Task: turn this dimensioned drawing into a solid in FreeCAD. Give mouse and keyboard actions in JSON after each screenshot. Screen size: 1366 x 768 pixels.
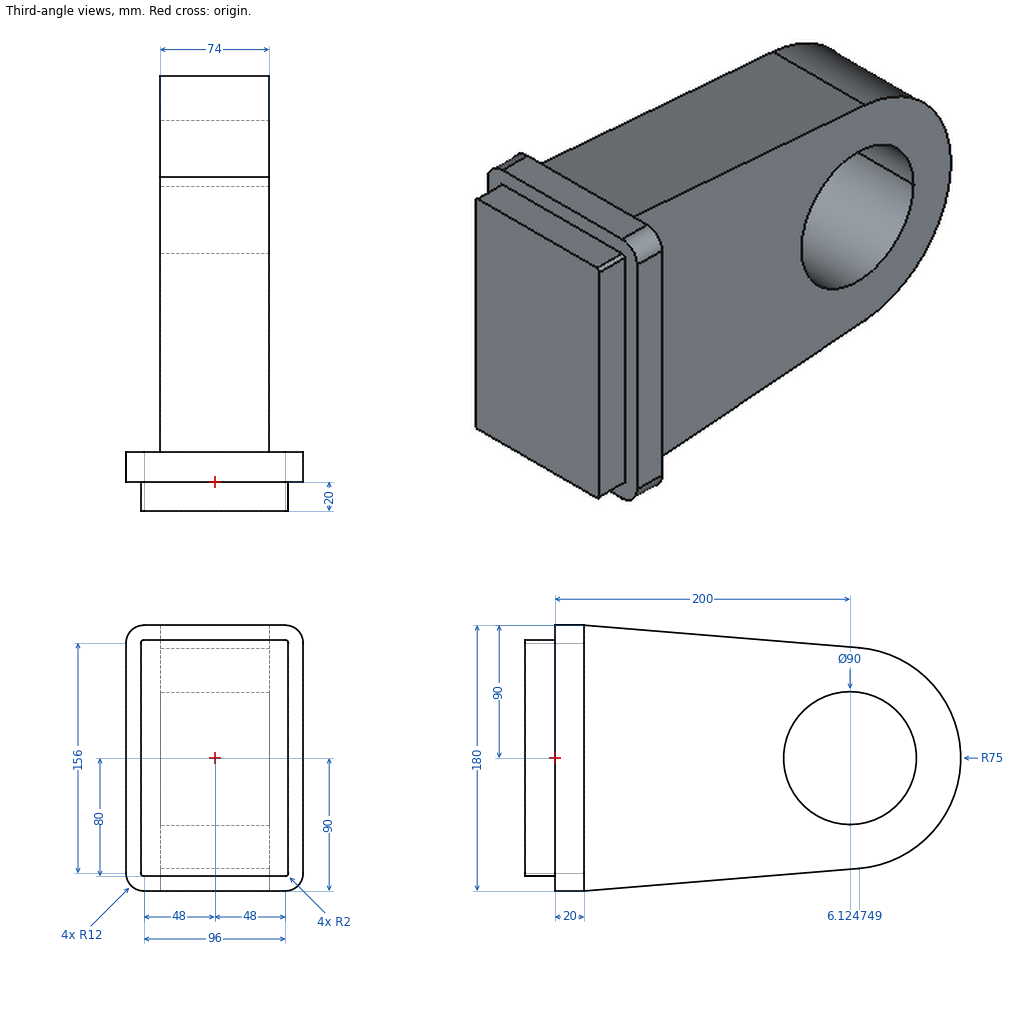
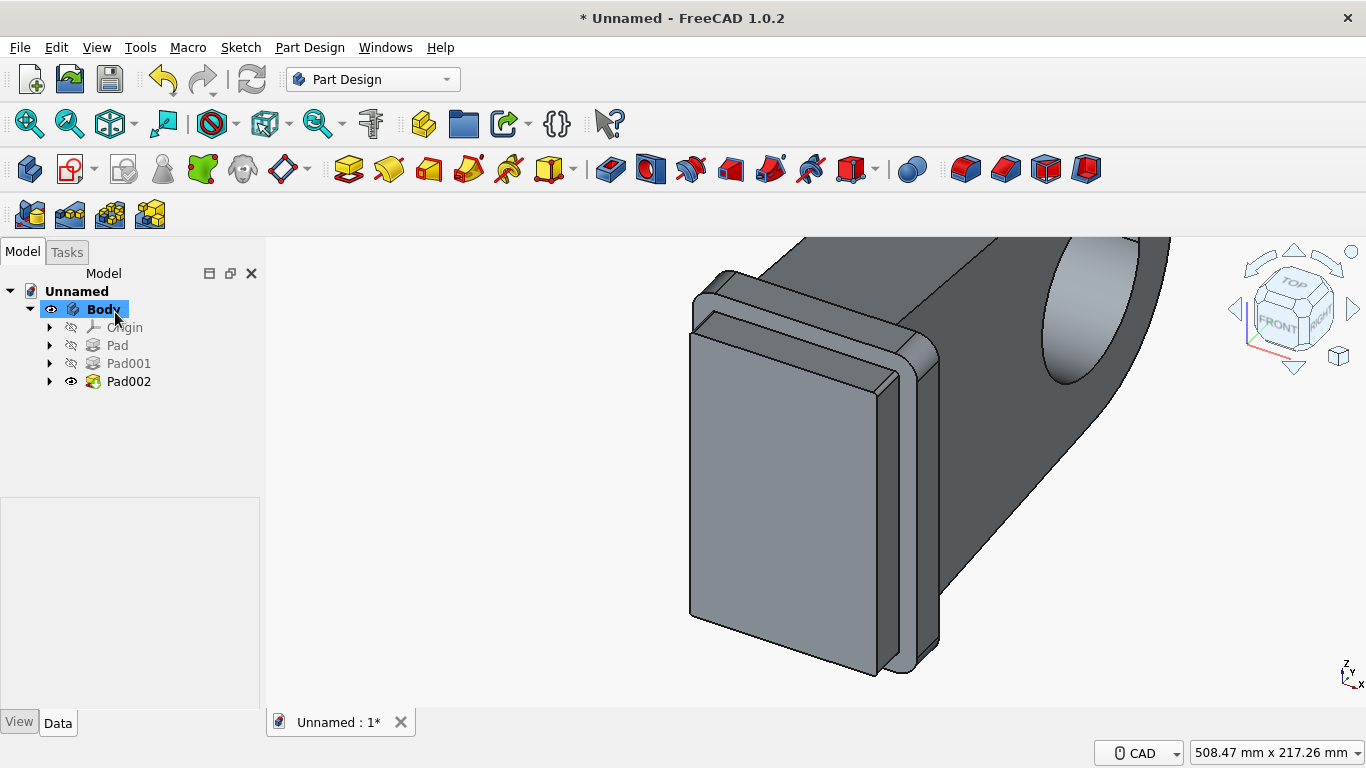
{"action": "key", "text": "0"}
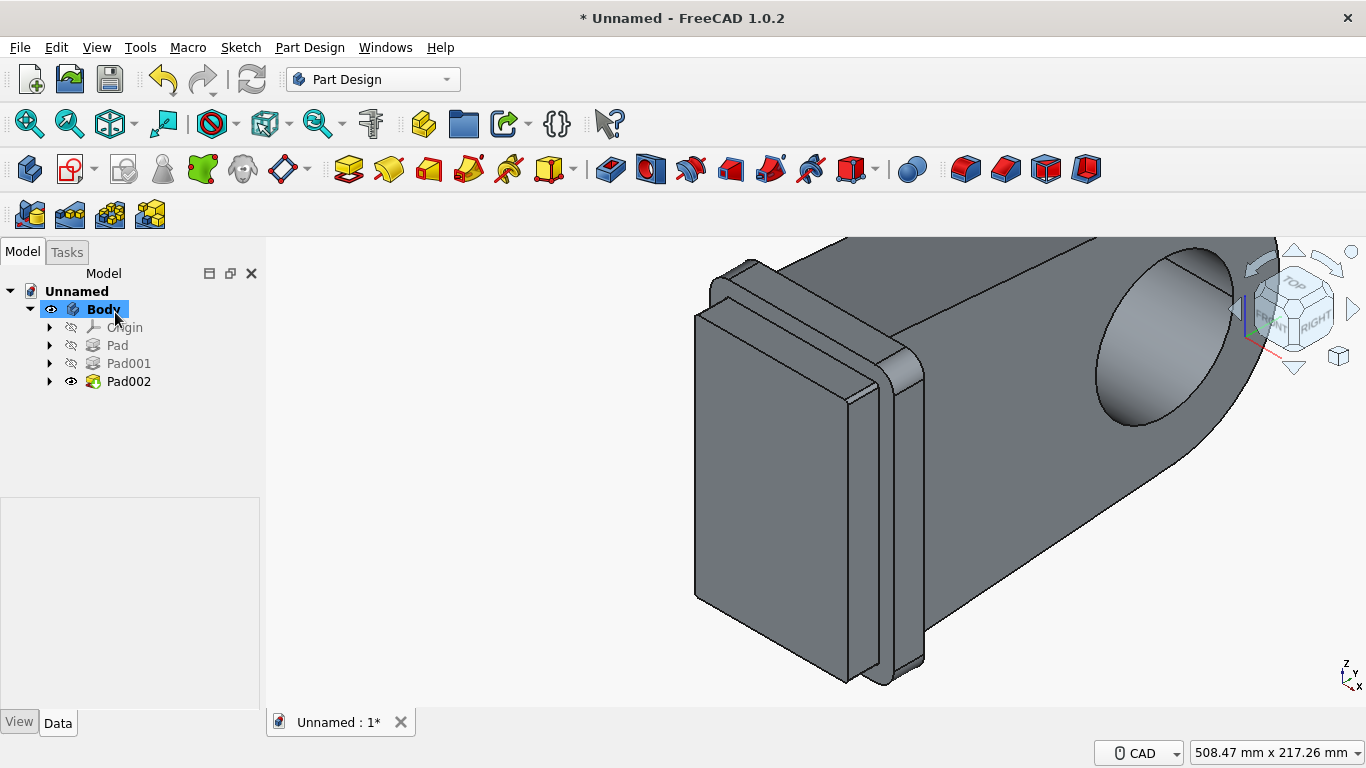
{"action": "left_click", "coordinate": [30, 124]}